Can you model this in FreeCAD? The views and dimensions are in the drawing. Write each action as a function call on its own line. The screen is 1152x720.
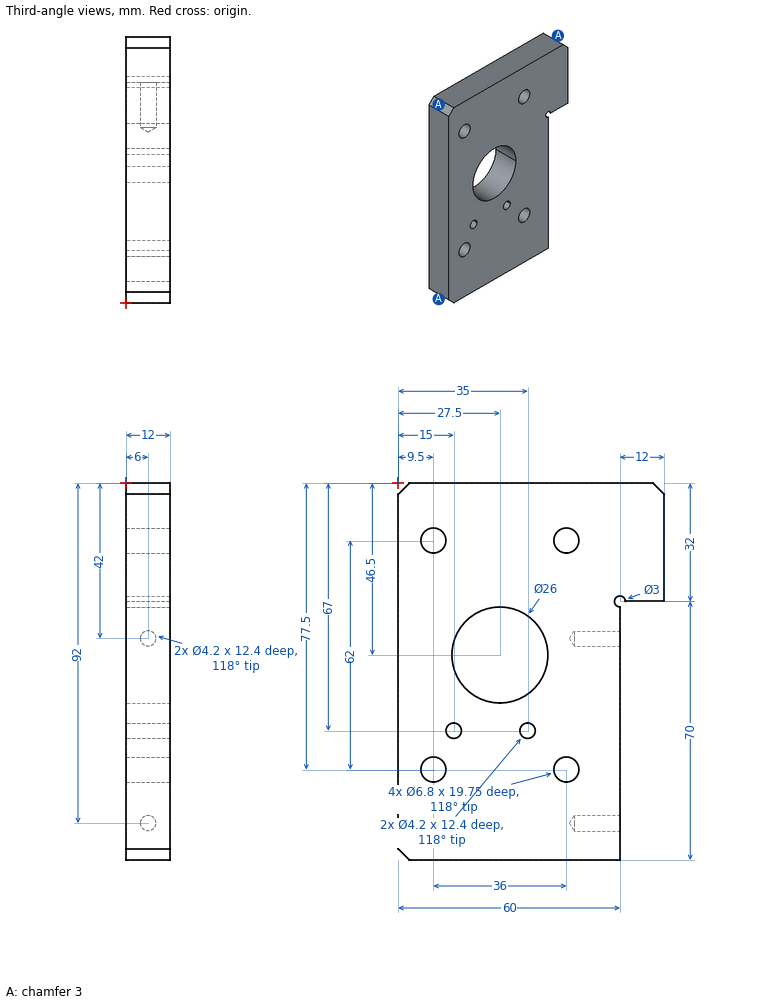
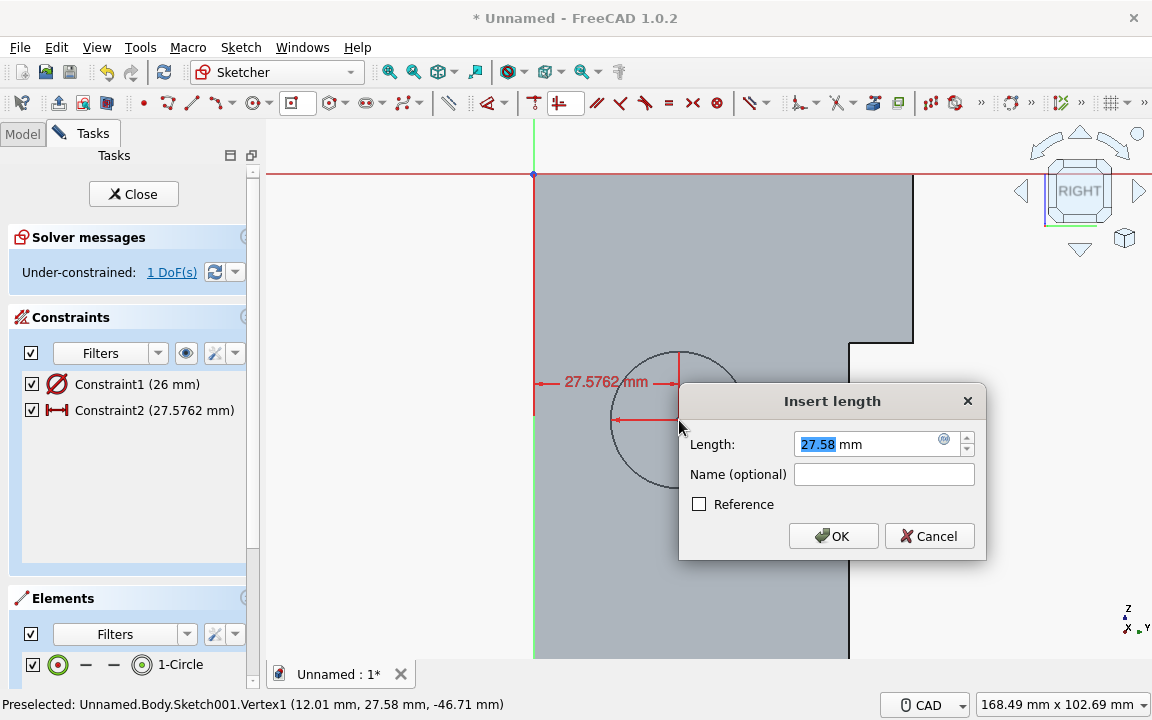
text(27.5)
key(Return)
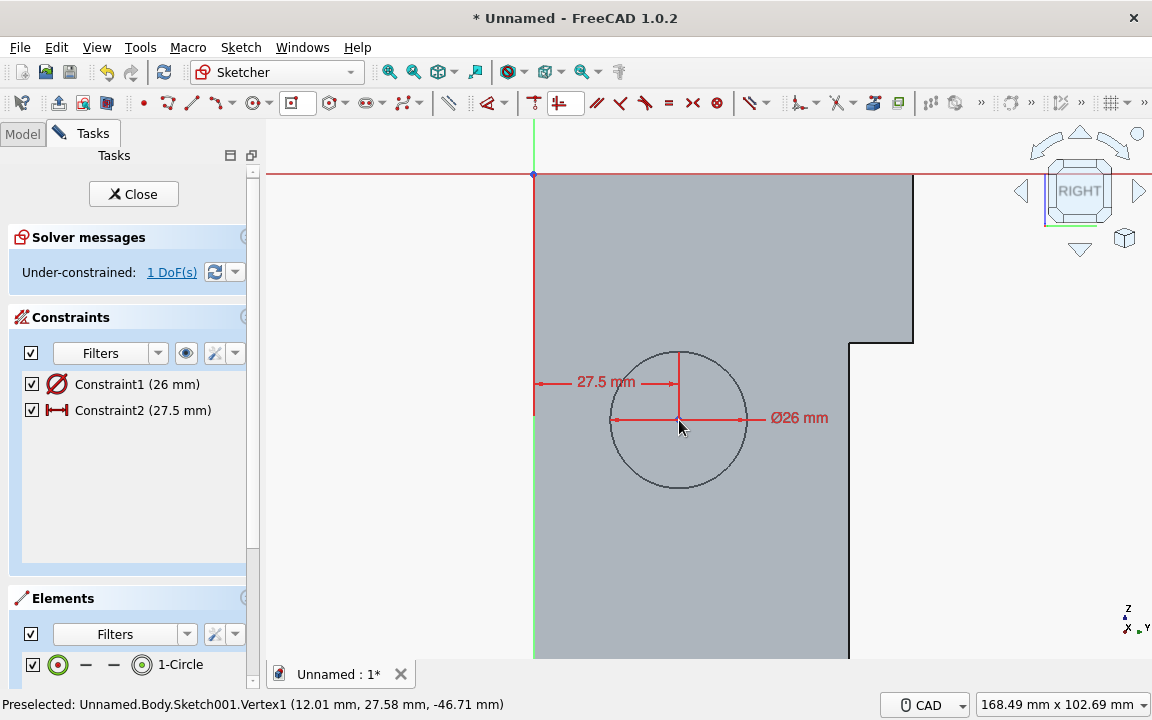
click(679, 420)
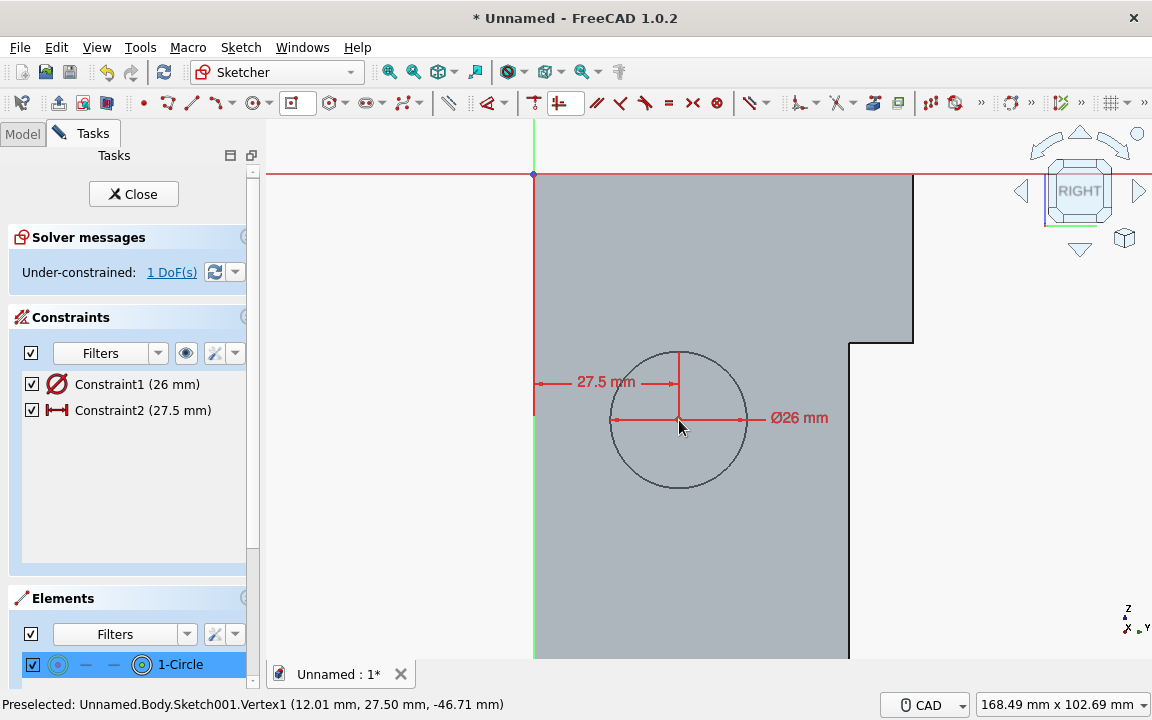
click(506, 104)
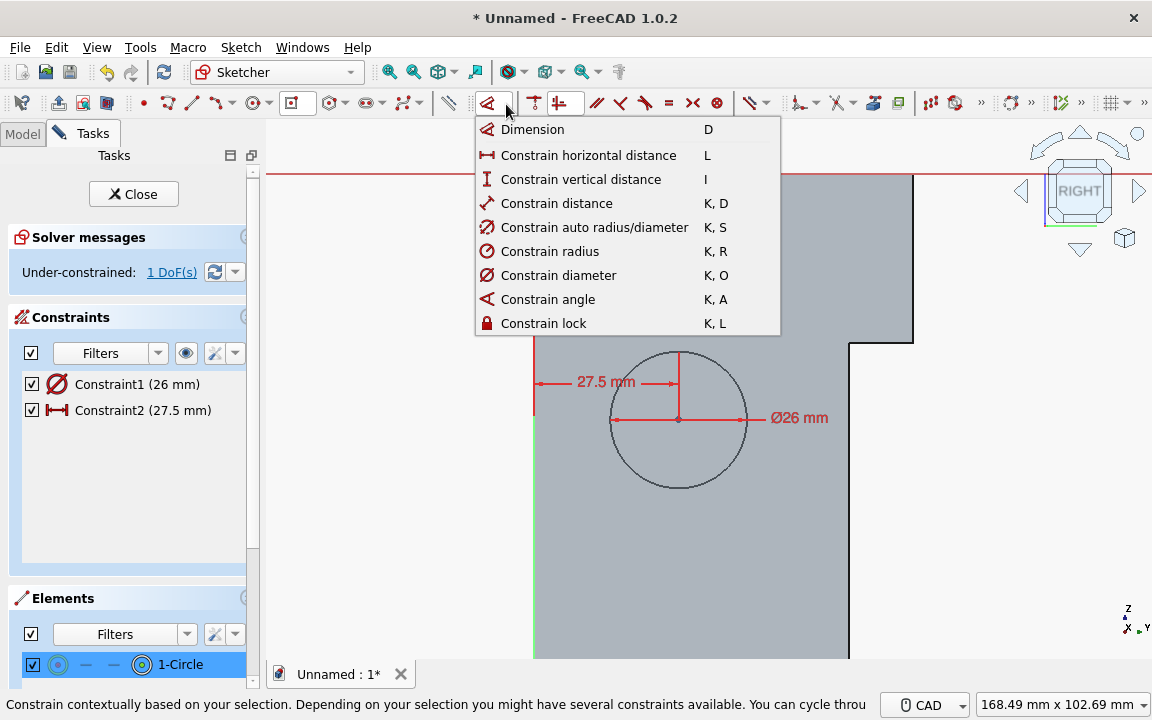
click(628, 179)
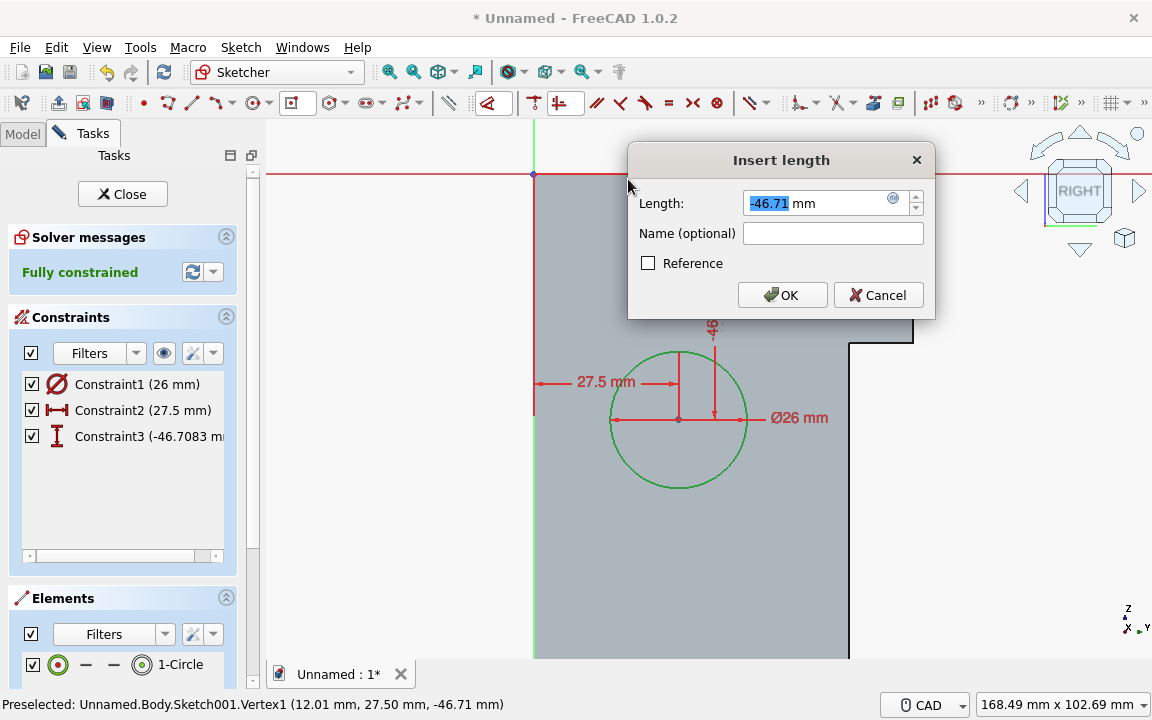
text(-46.5)
key(Return)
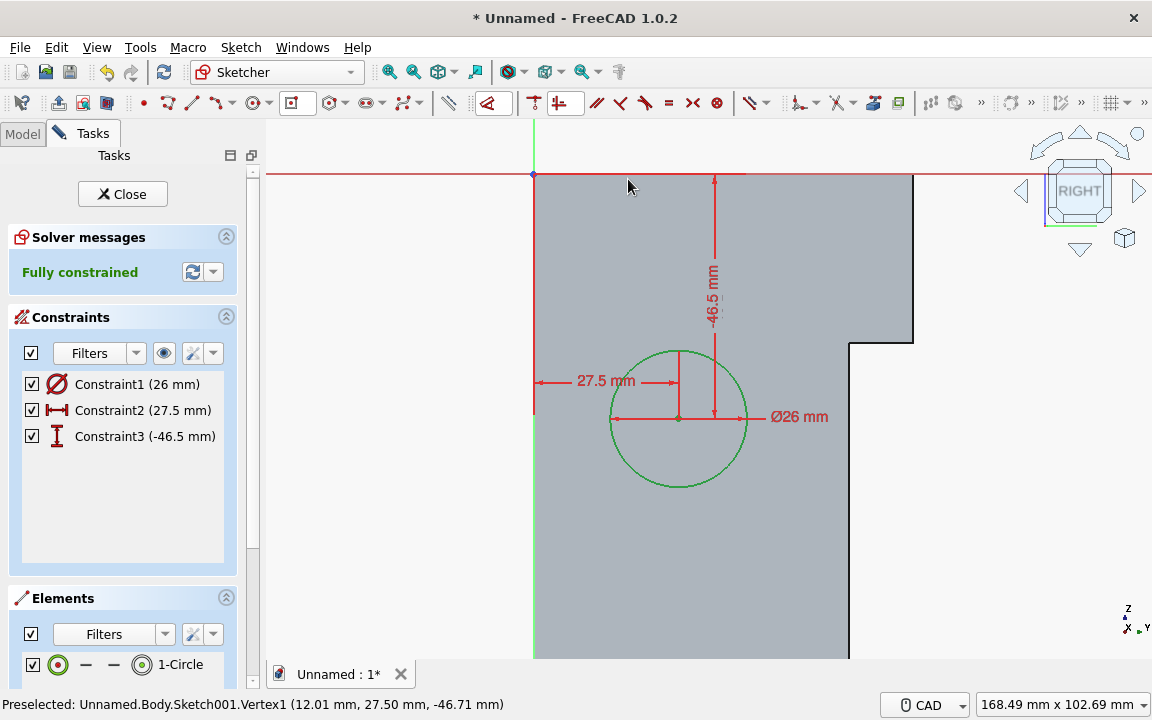
click(123, 194)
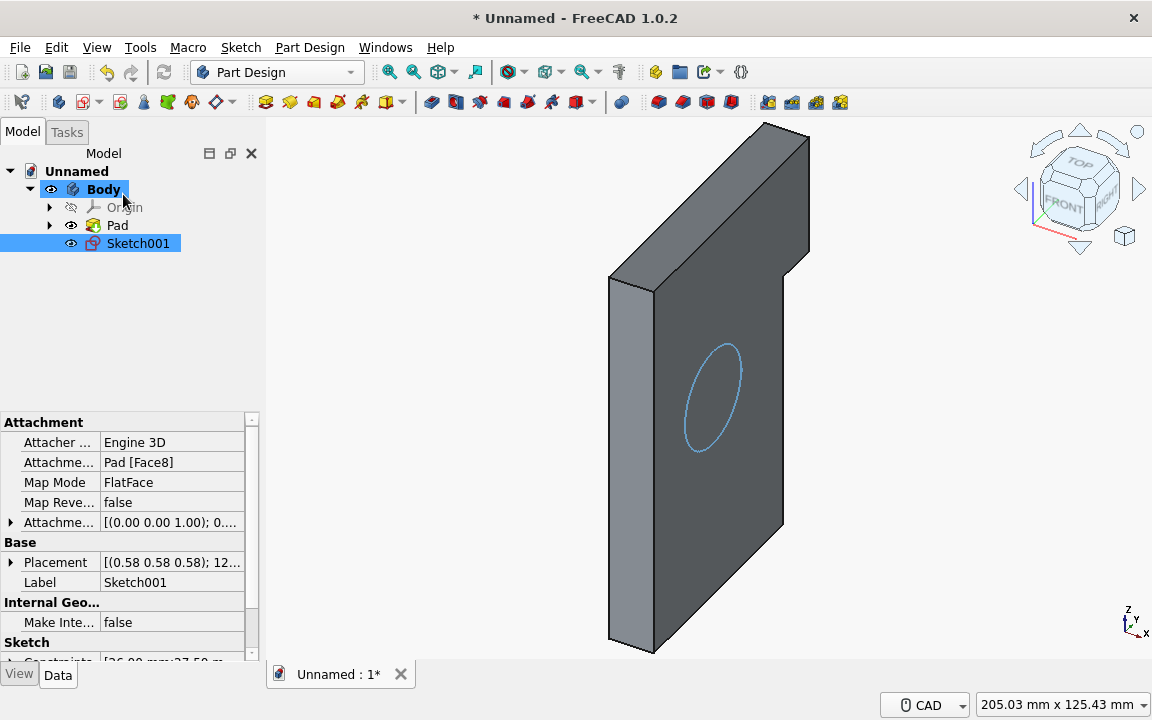
click(432, 102)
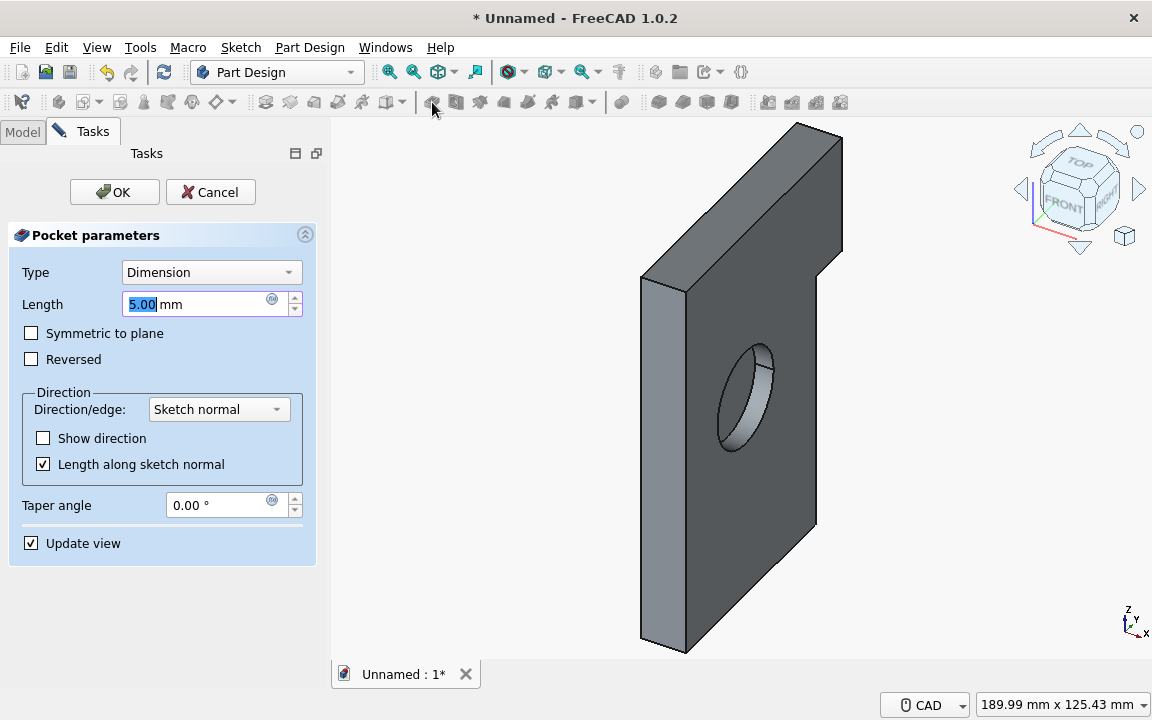
click(212, 272)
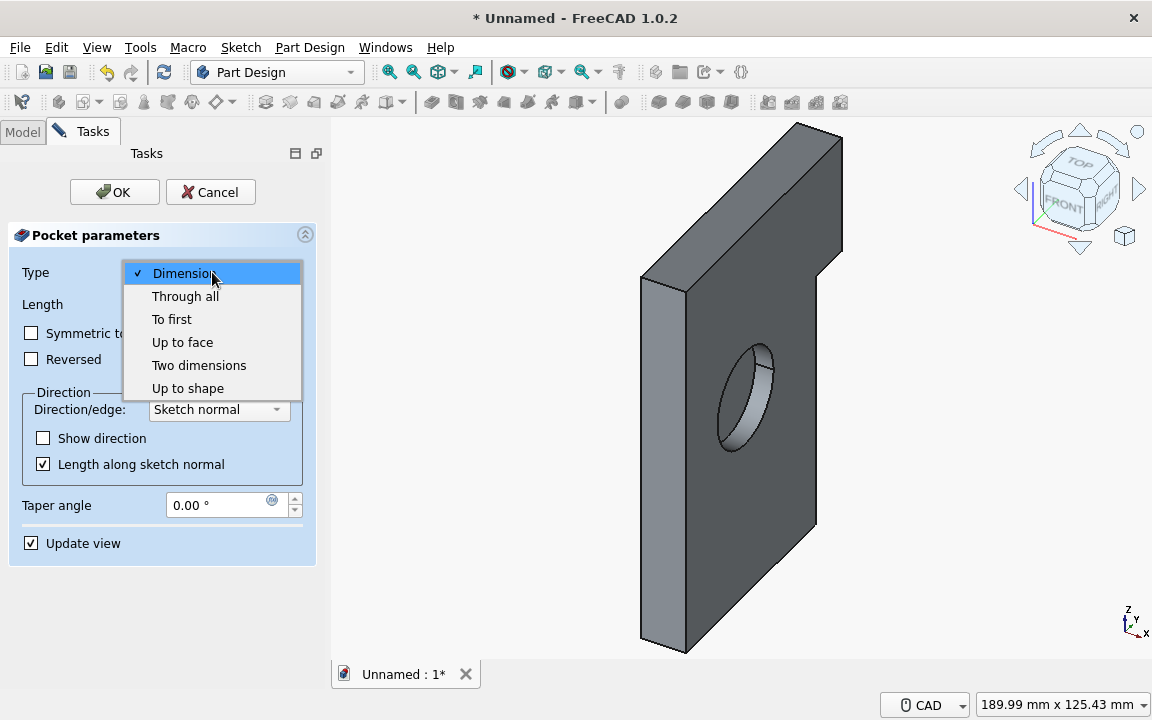
click(212, 296)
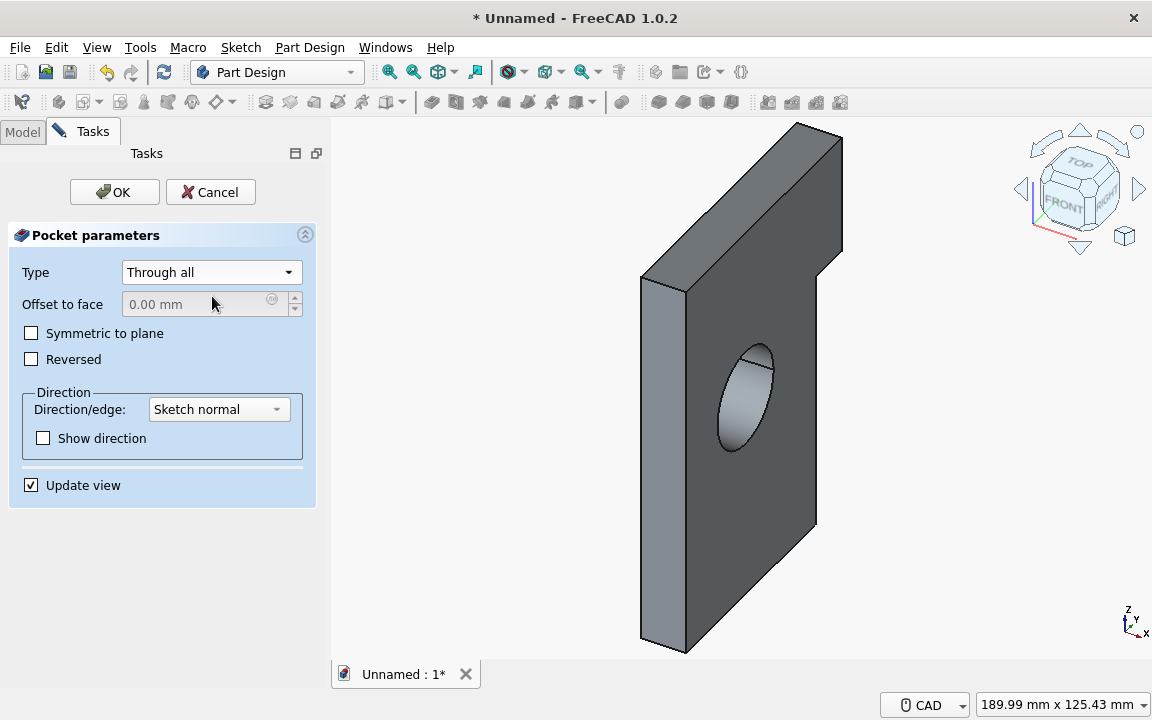
click(115, 192)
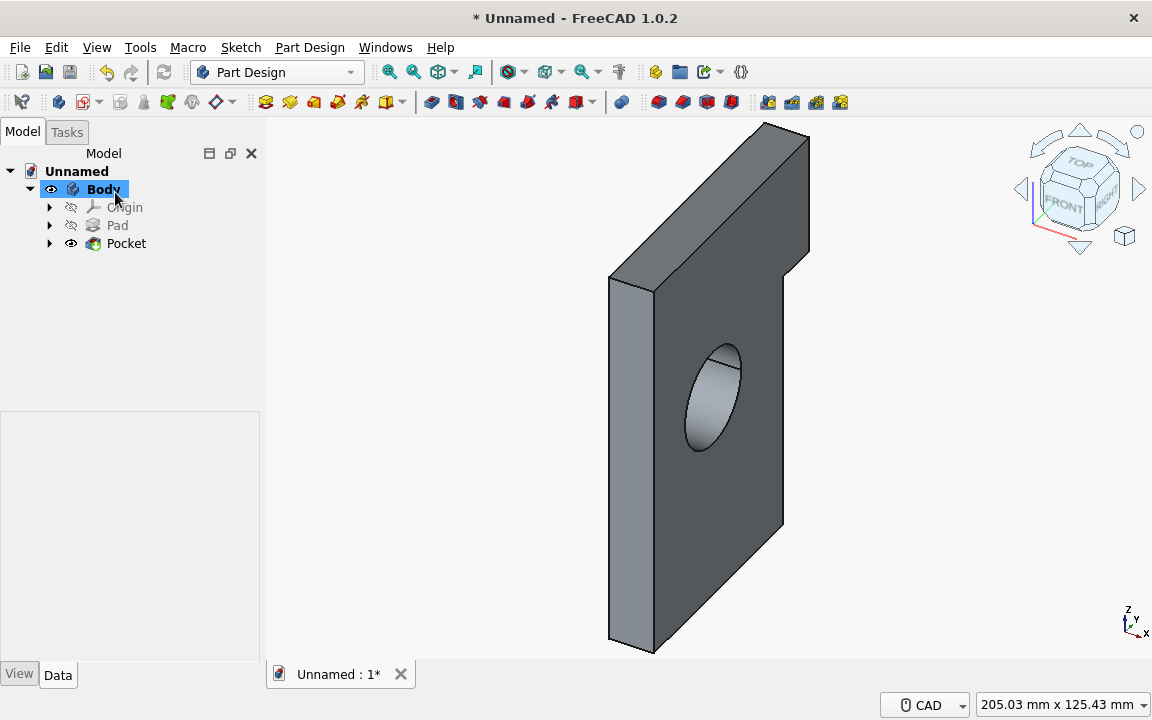
click(84, 102)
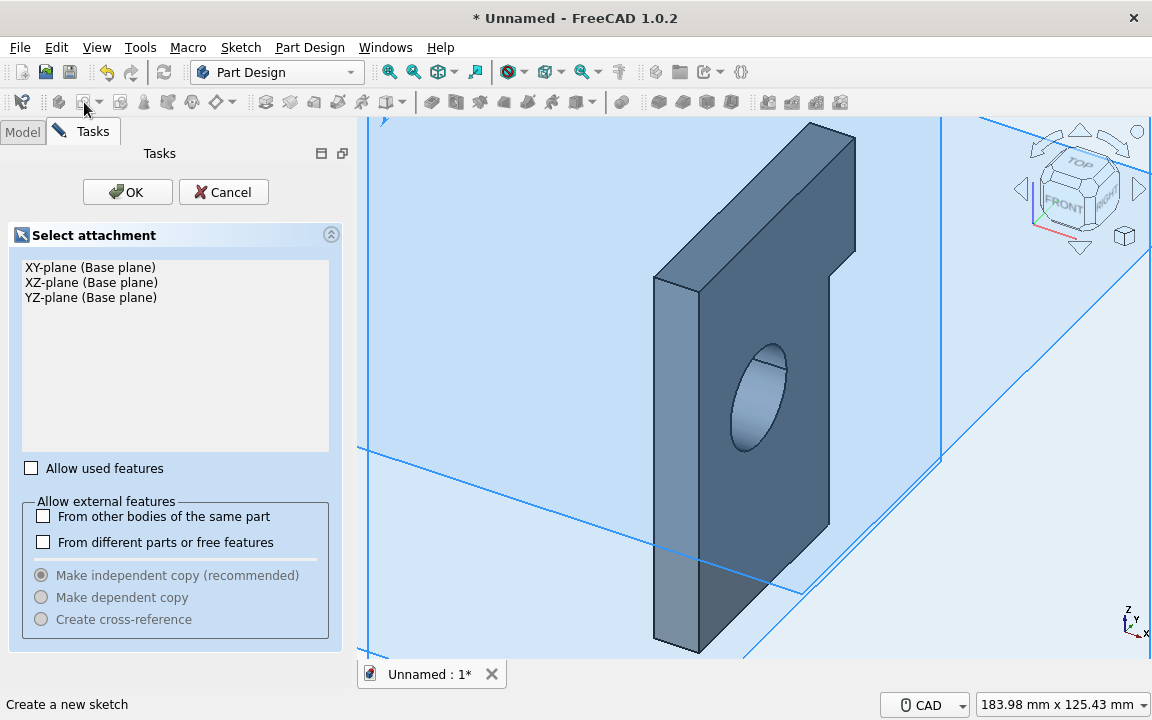
click(82, 298)